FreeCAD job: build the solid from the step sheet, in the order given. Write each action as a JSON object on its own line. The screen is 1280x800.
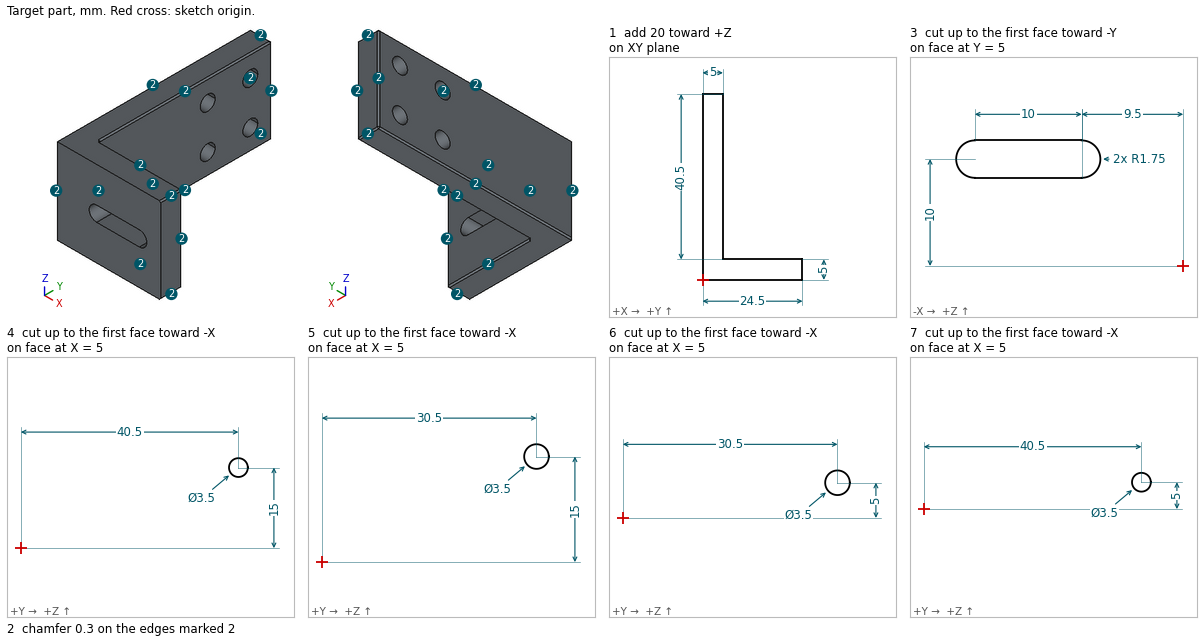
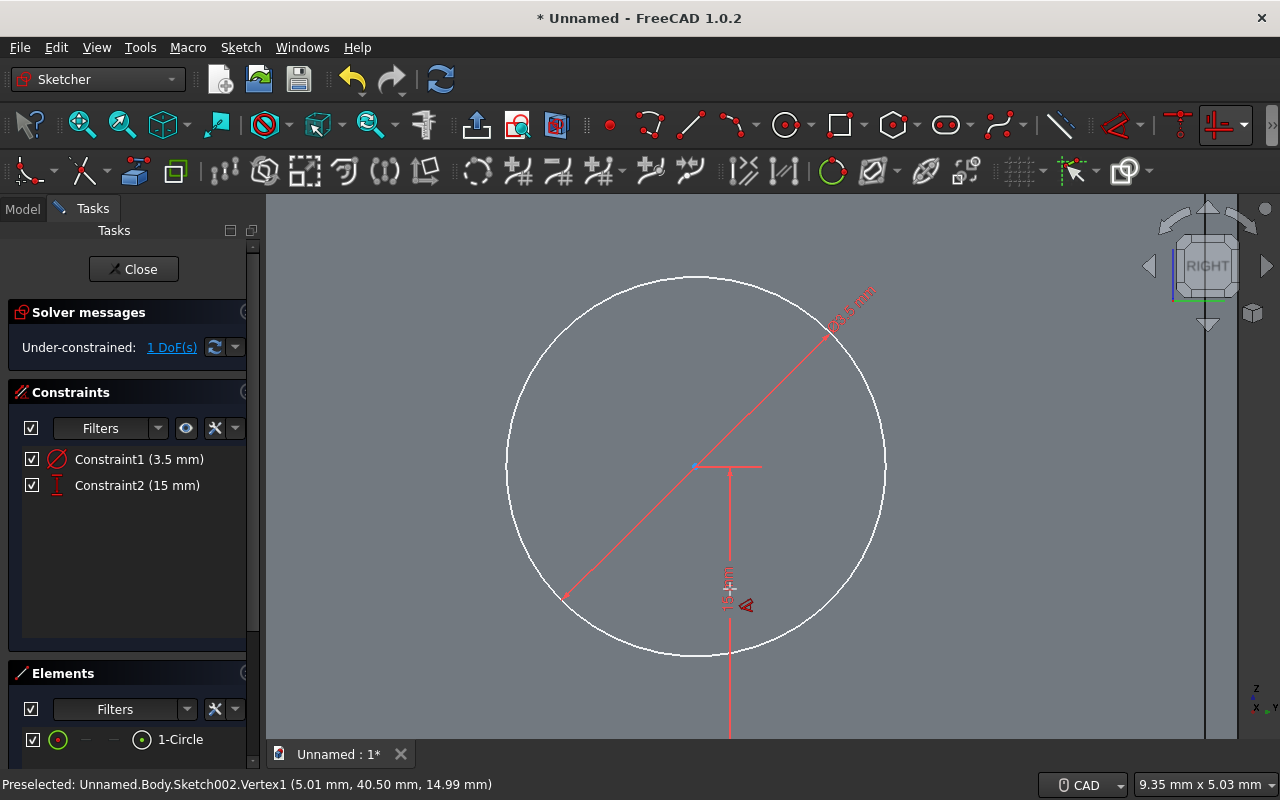
{"action": "left_click", "coordinate": [696, 467]}
{"action": "left_click", "coordinate": [495, 433]}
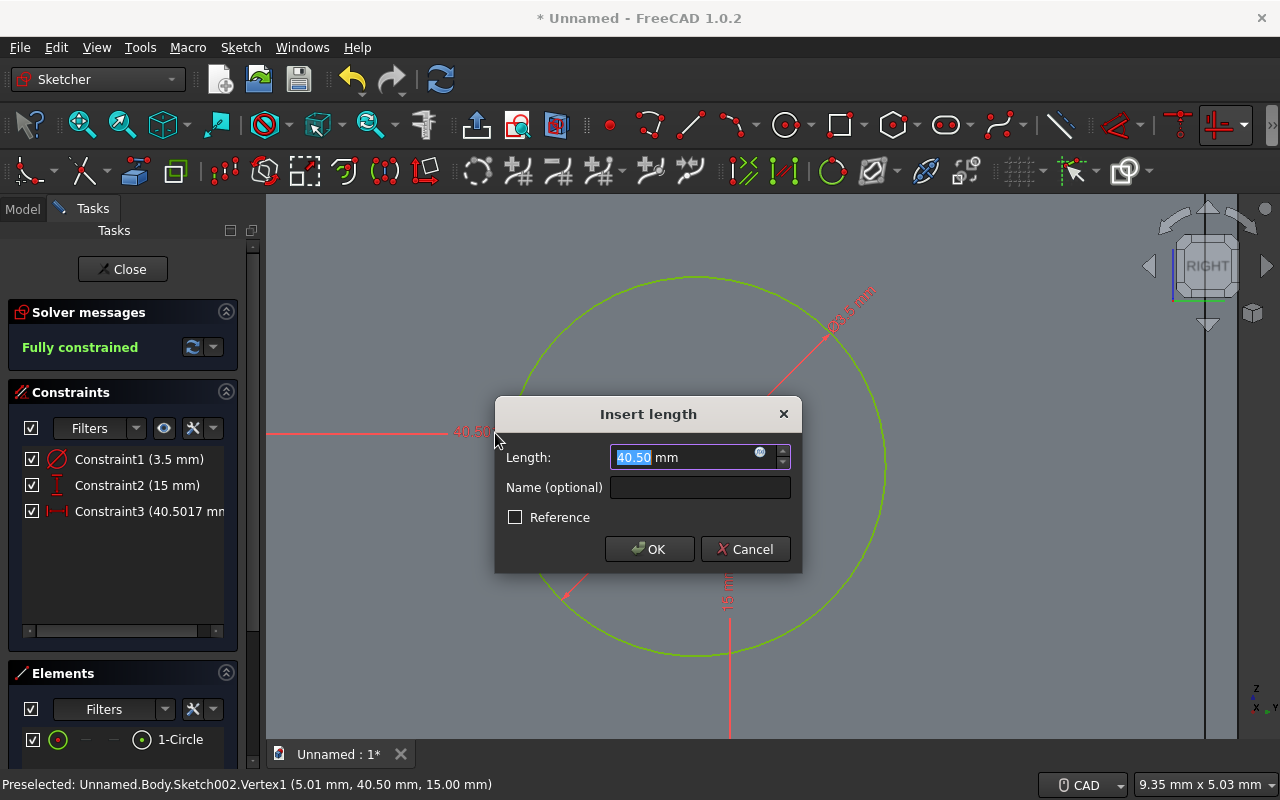
{"action": "type", "text": "40.5"}
{"action": "key", "text": "Return"}
{"action": "key", "text": "Escape"}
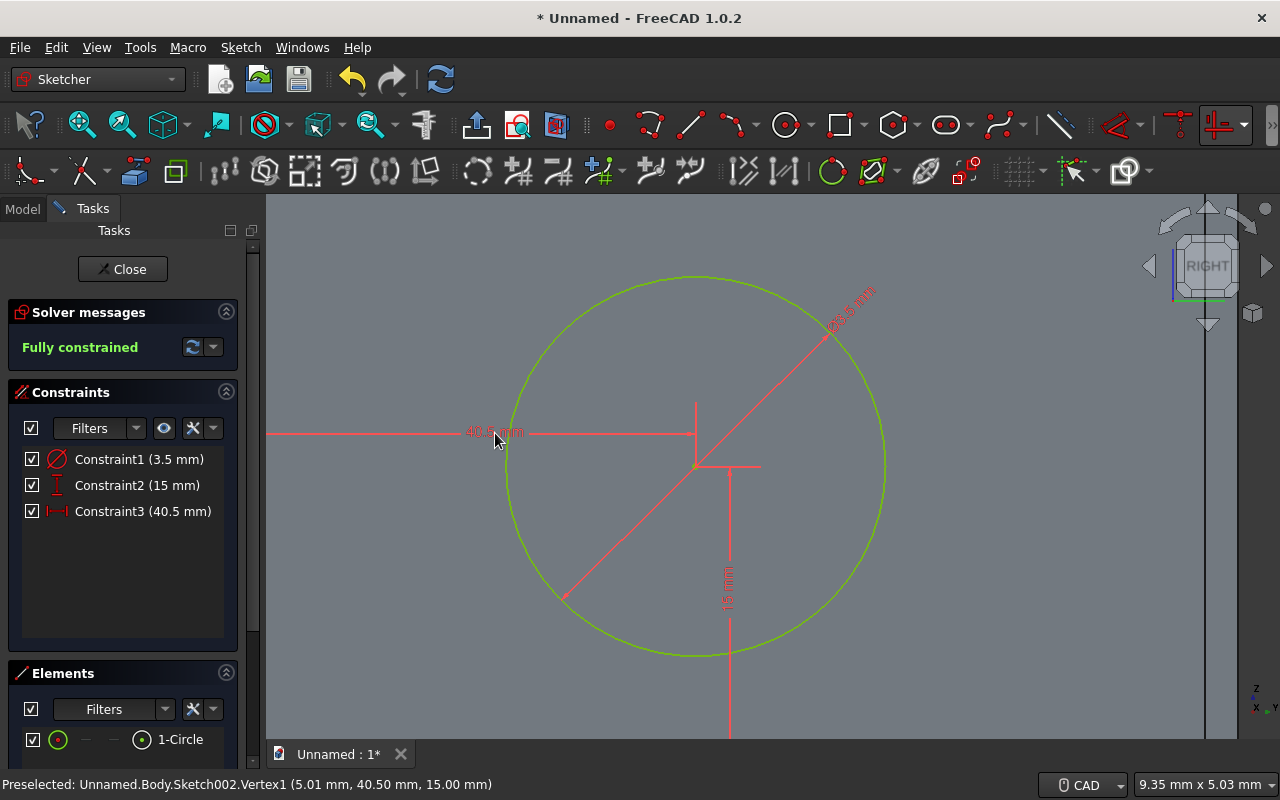
{"action": "left_click", "coordinate": [123, 269]}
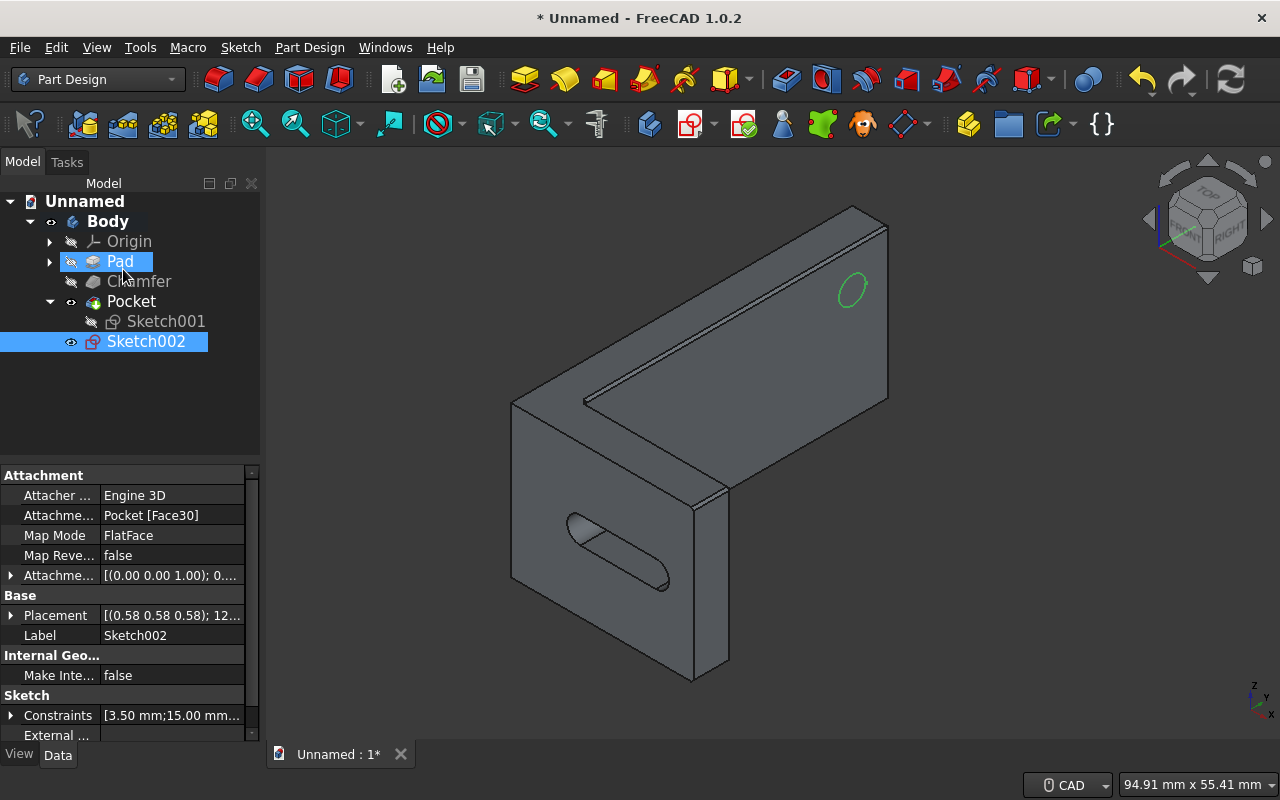
{"action": "left_click", "coordinate": [788, 80]}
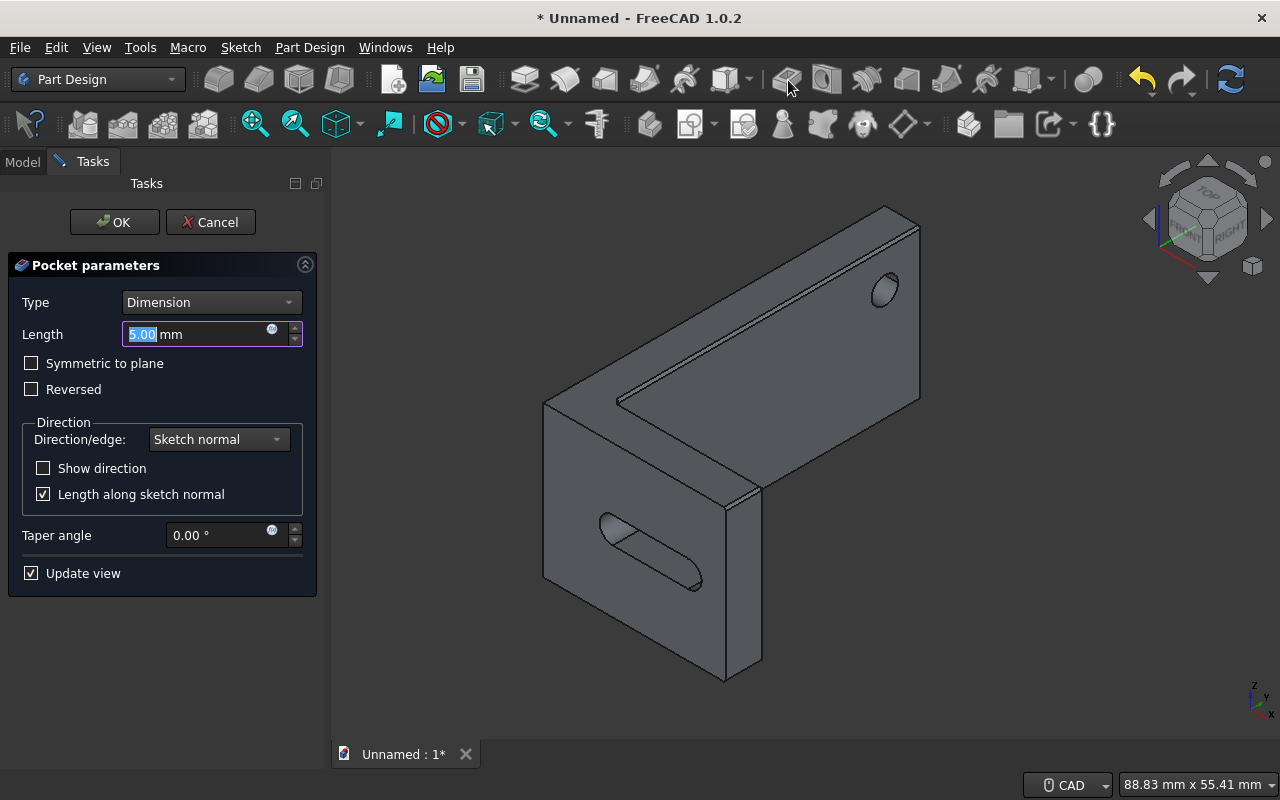
{"action": "left_click", "coordinate": [212, 302]}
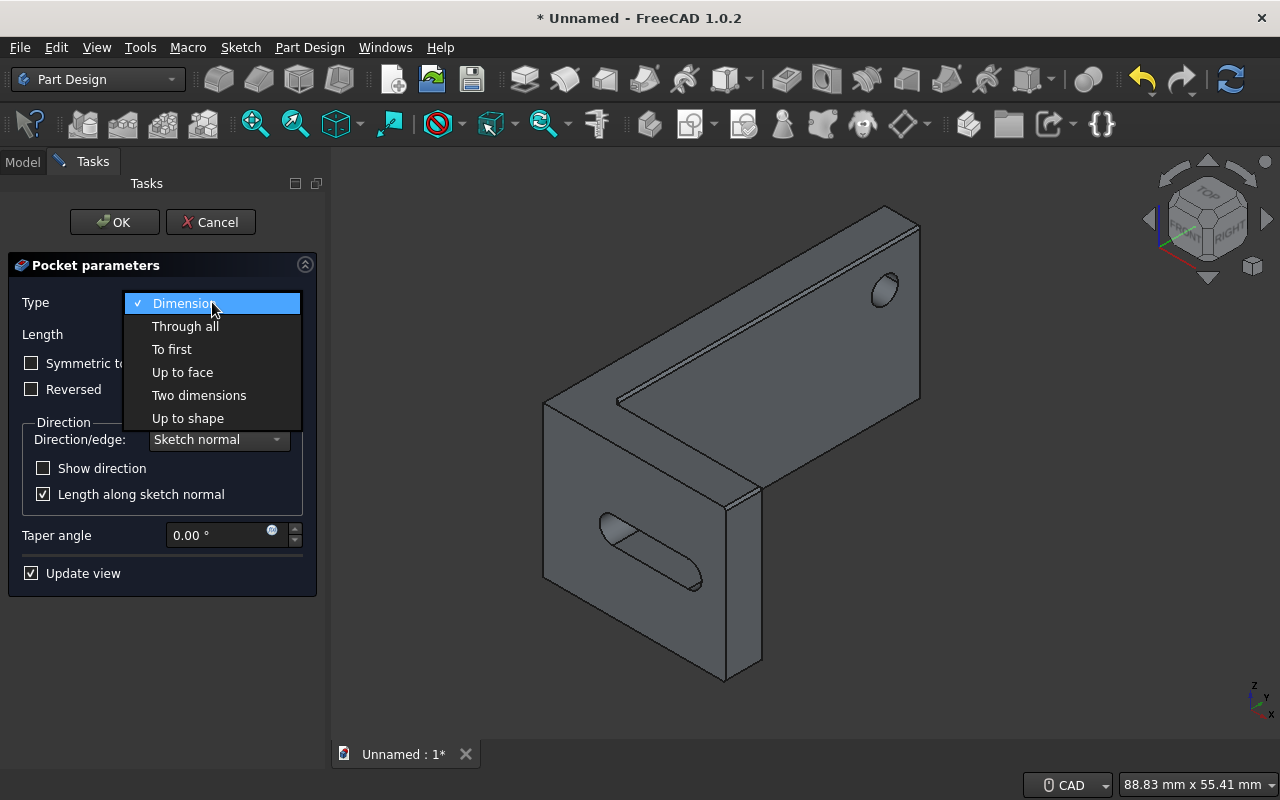
{"action": "left_click", "coordinate": [212, 350]}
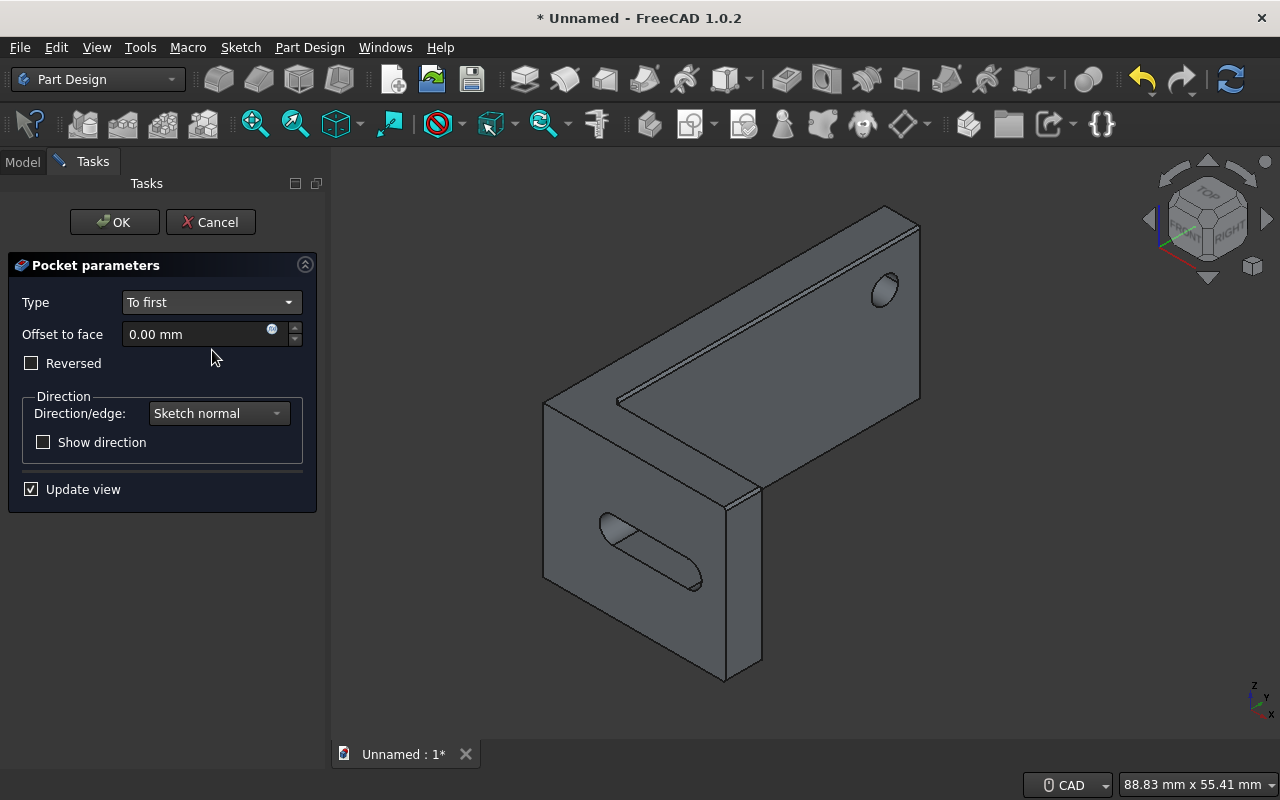
{"action": "left_click", "coordinate": [115, 222]}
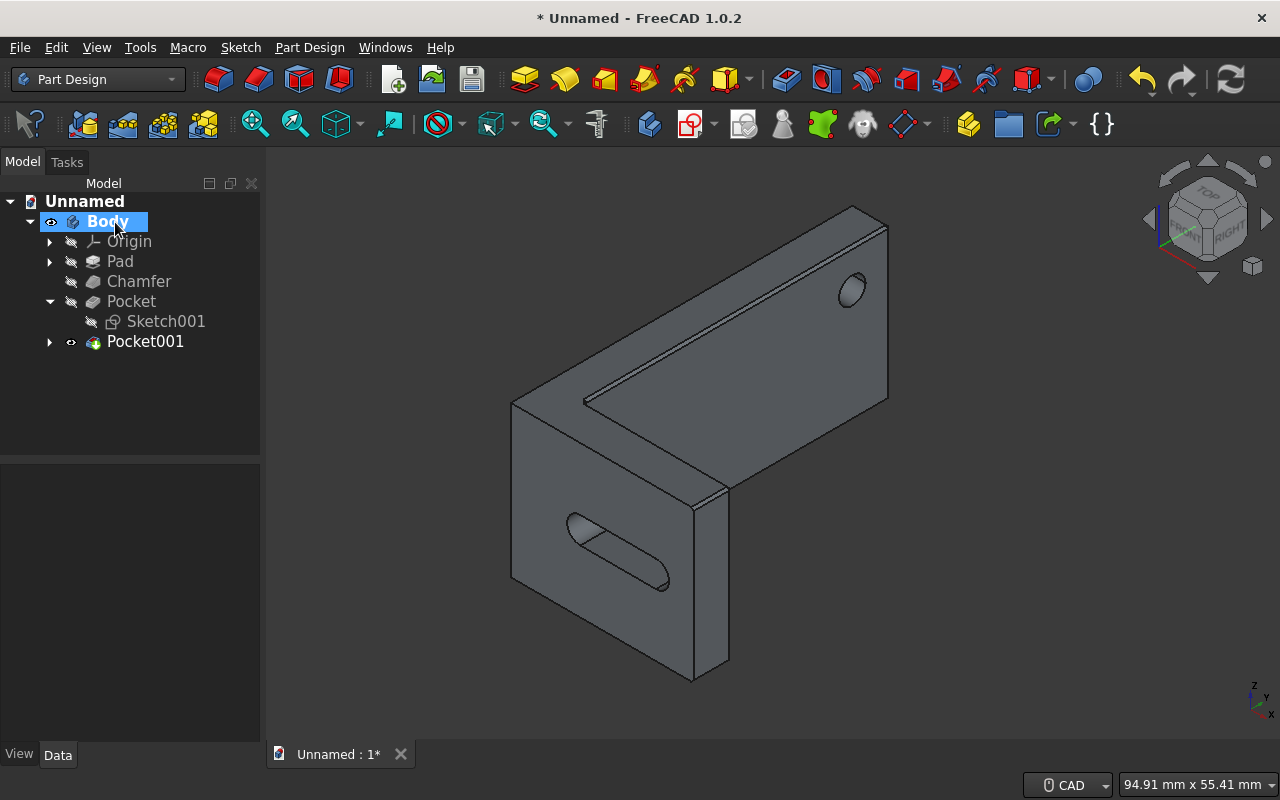
{"action": "left_click", "coordinate": [737, 399]}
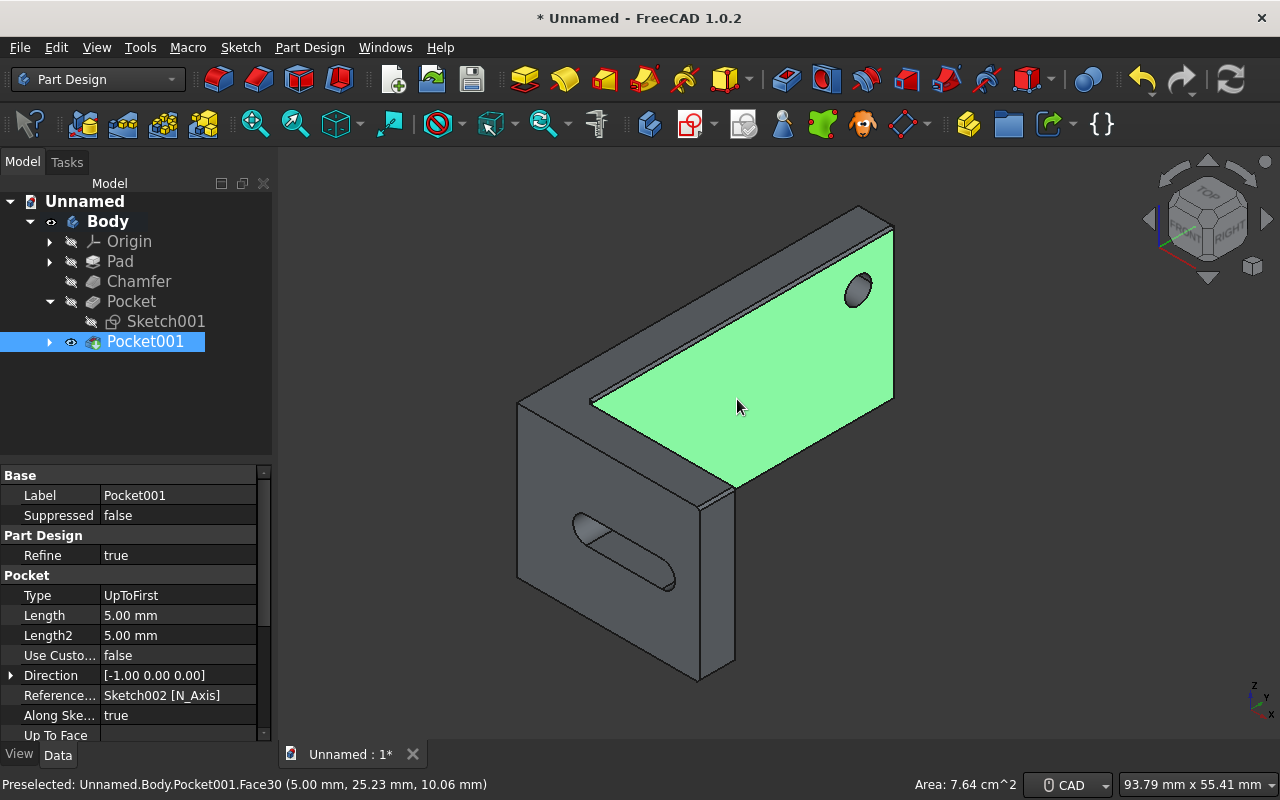
{"action": "left_click", "coordinate": [690, 124]}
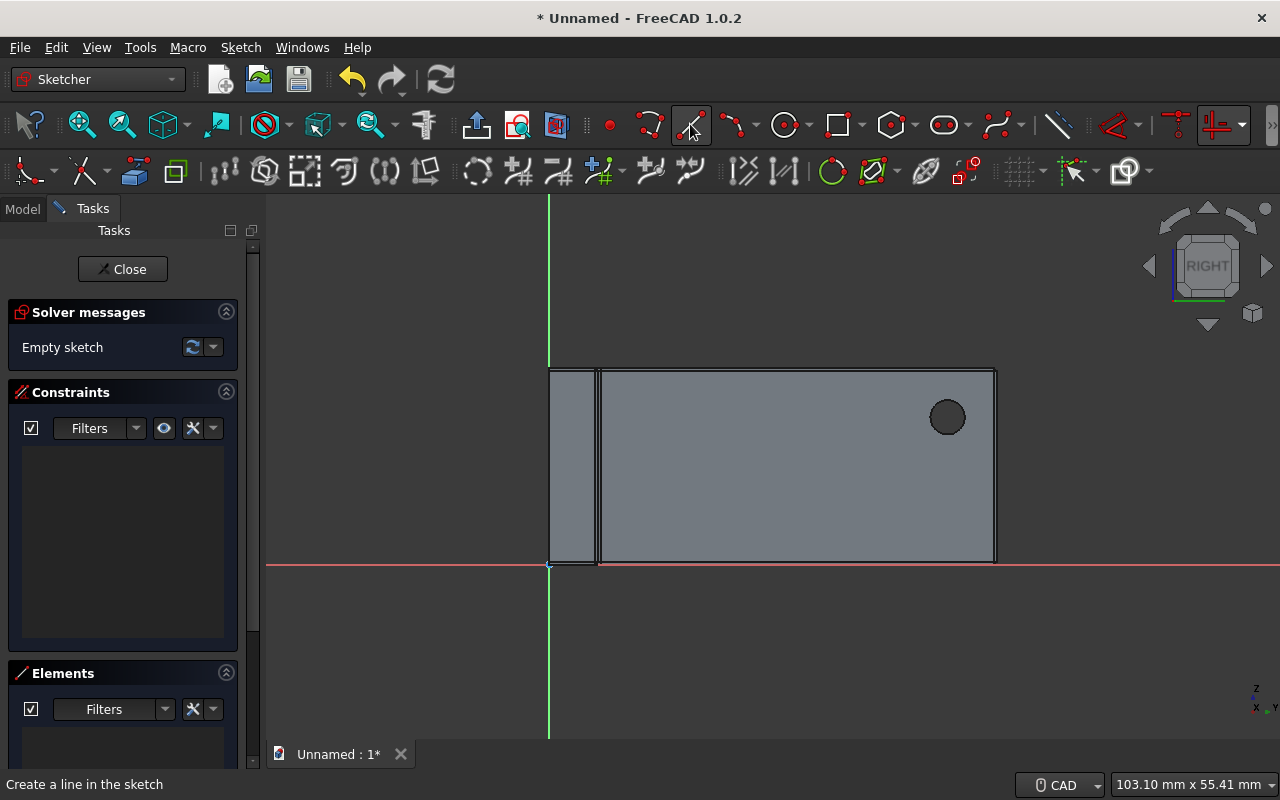
{"action": "scroll", "coordinate": [864, 412], "scroll_direction": "up", "scroll_amount": 12}